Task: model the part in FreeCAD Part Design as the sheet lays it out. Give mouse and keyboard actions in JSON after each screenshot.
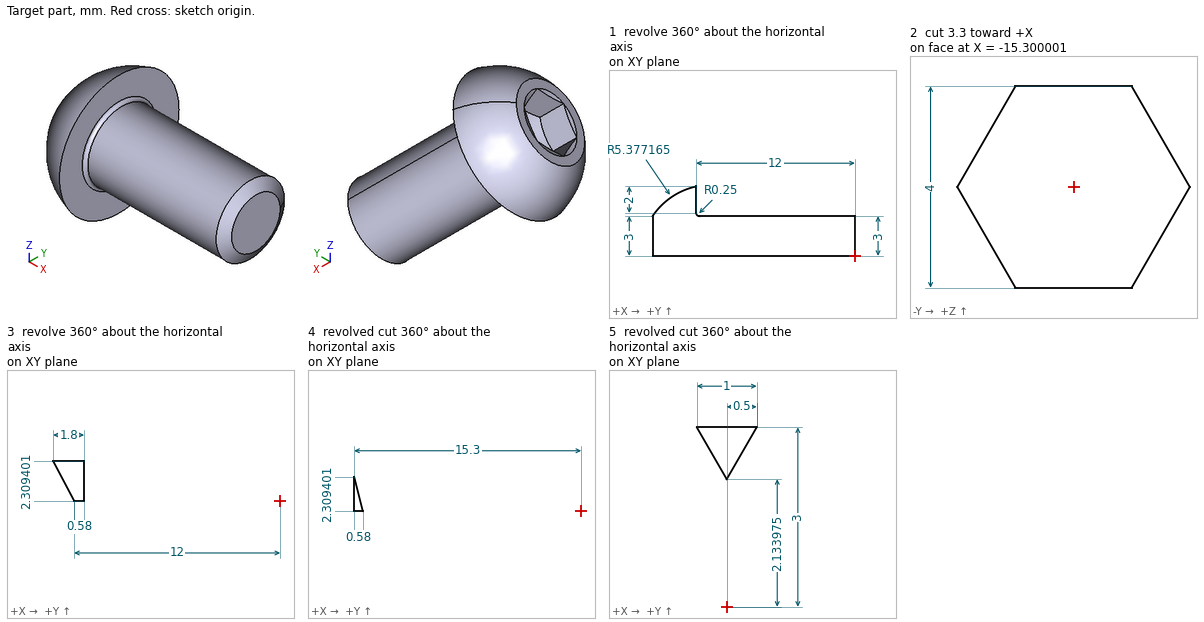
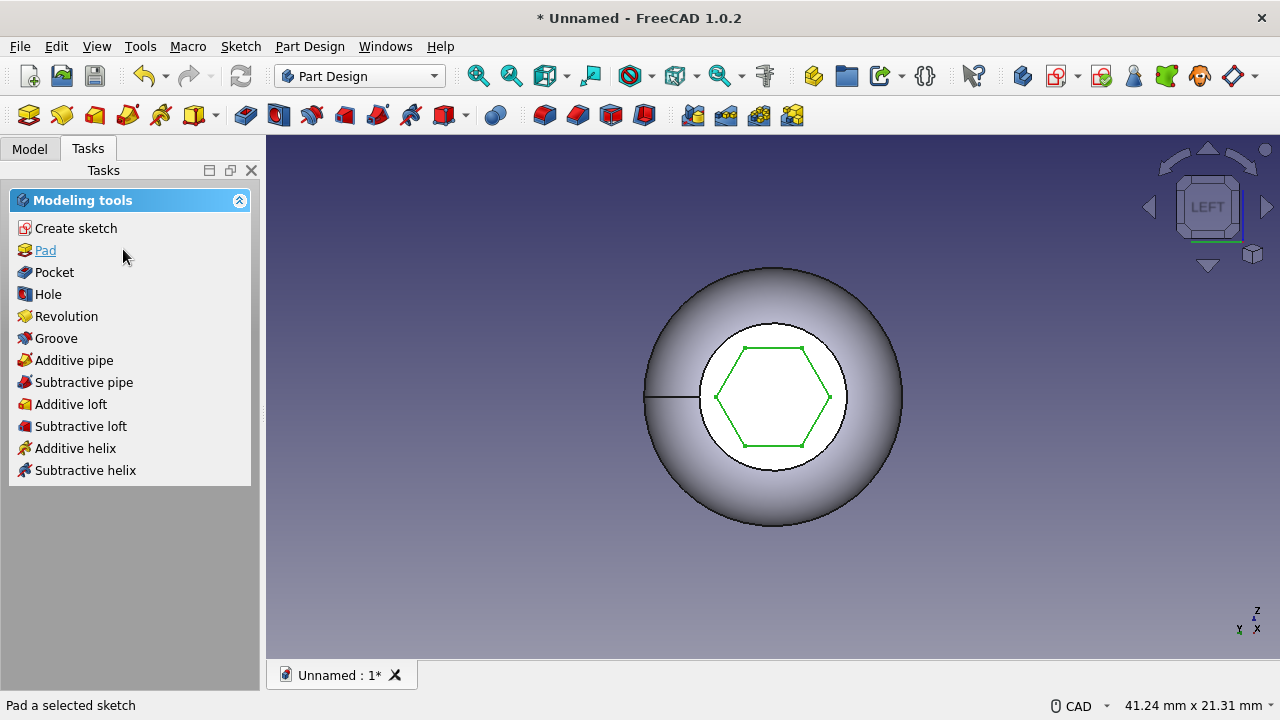
{"action": "left_click", "coordinate": [246, 116]}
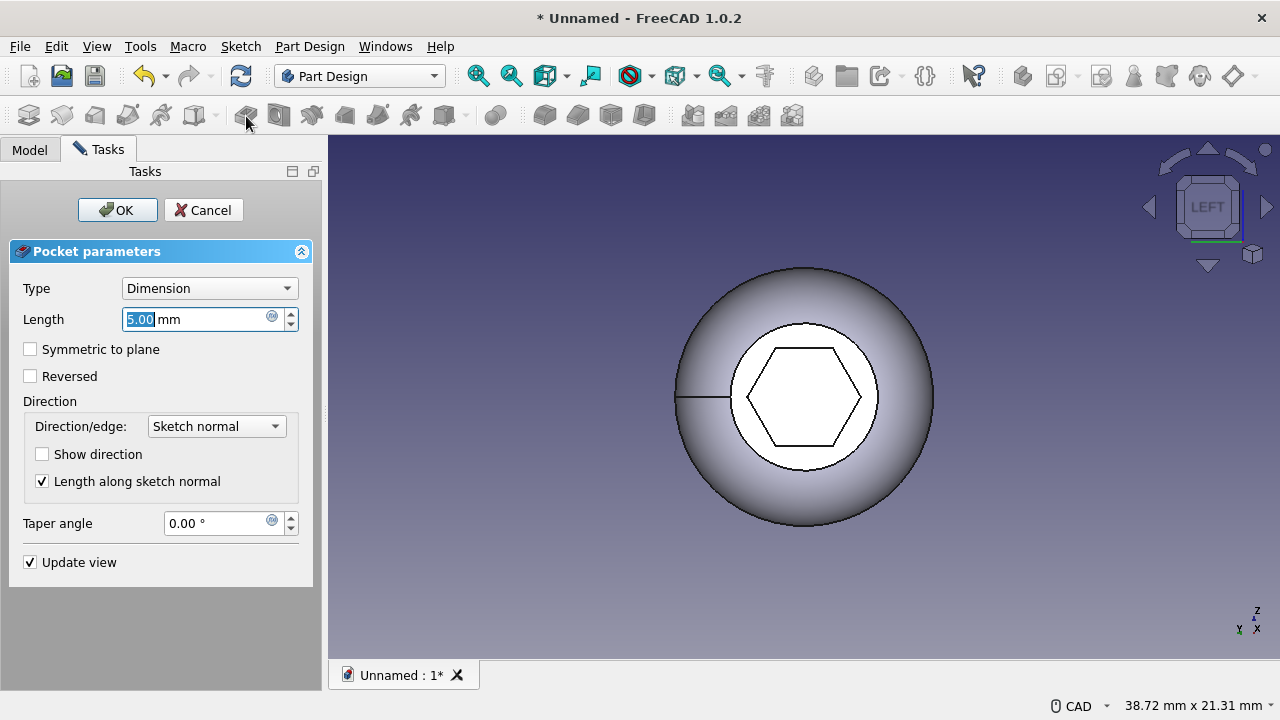
{"action": "type", "text": "3.3"}
{"action": "key", "text": "Tab"}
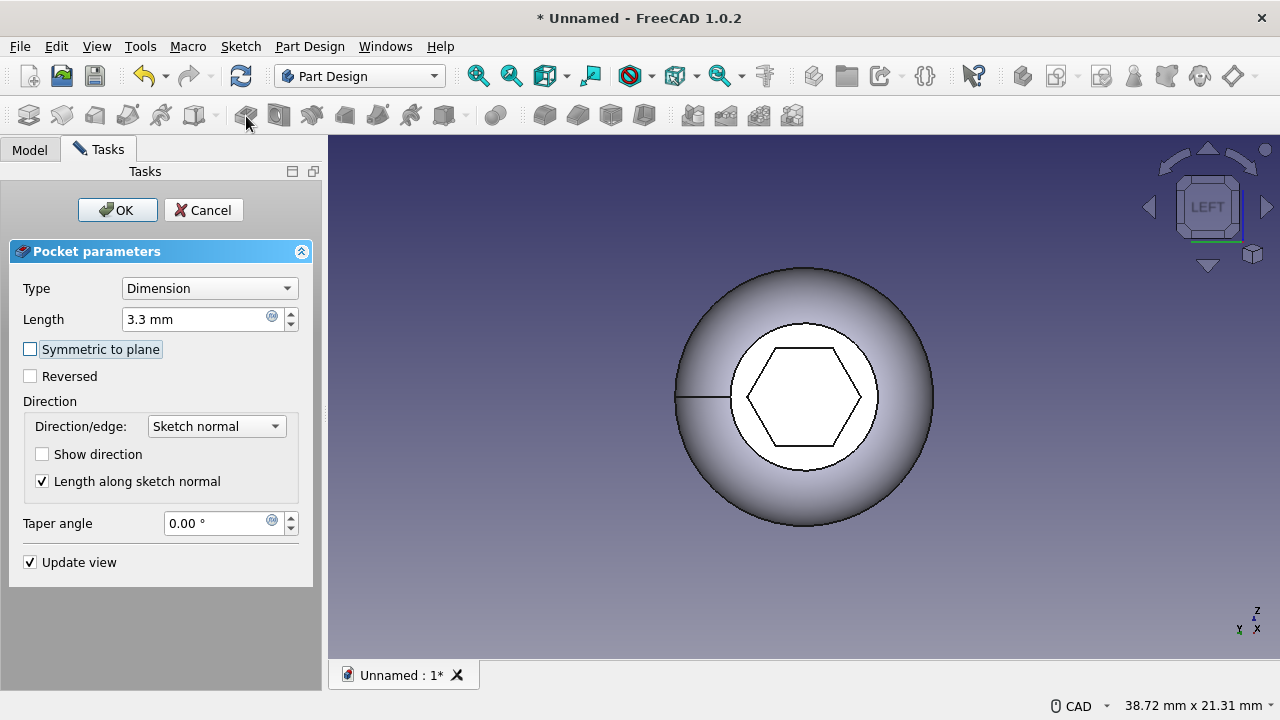
{"action": "left_click", "coordinate": [118, 210]}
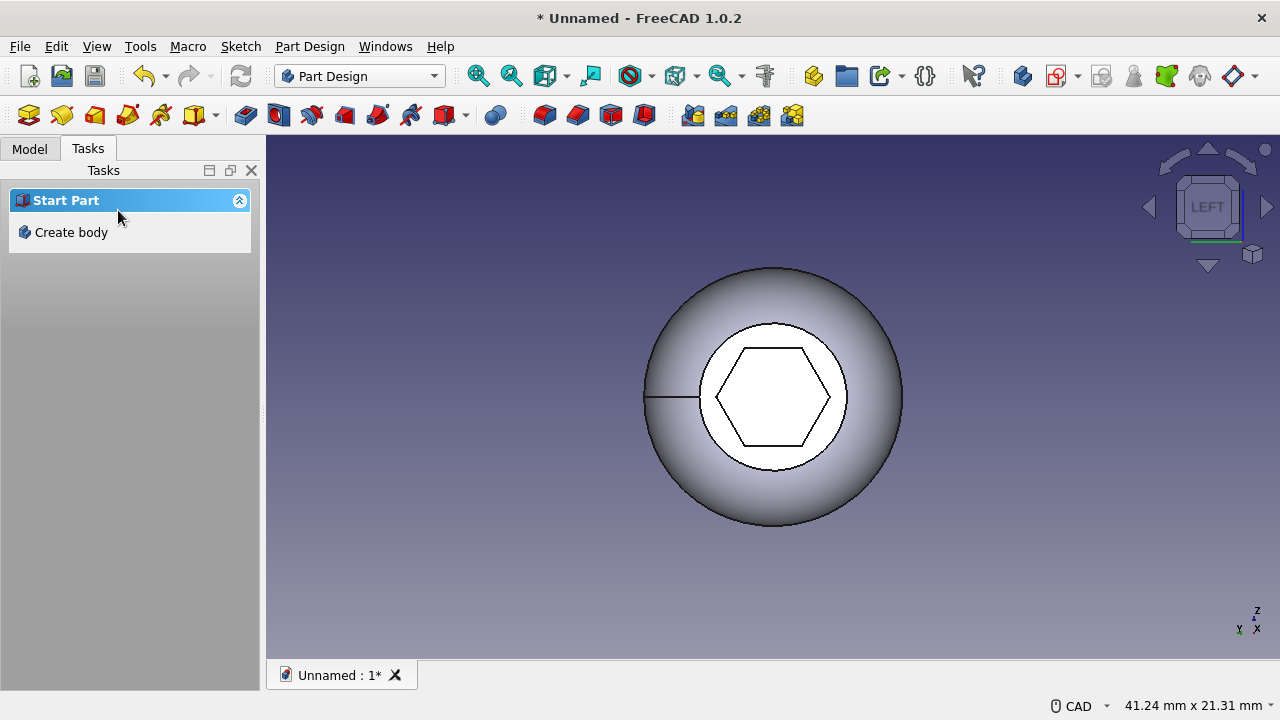
{"action": "left_click", "coordinate": [1056, 76]}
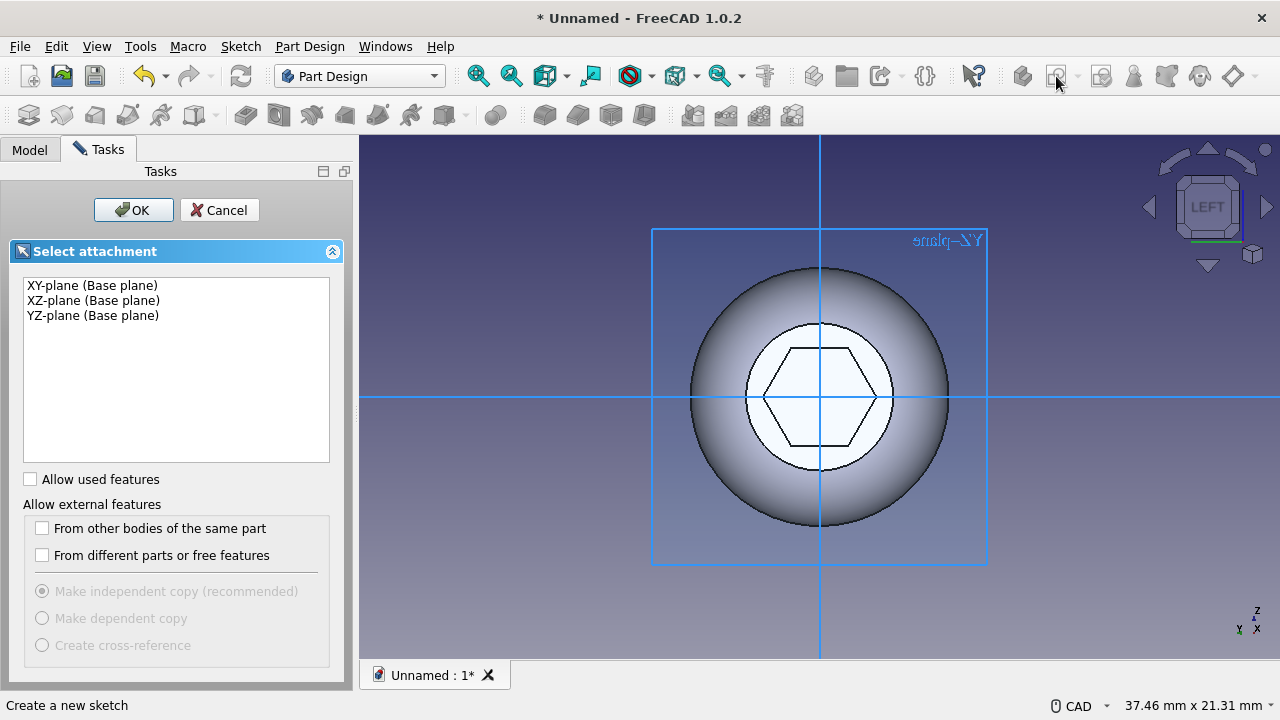
{"action": "left_click", "coordinate": [84, 286]}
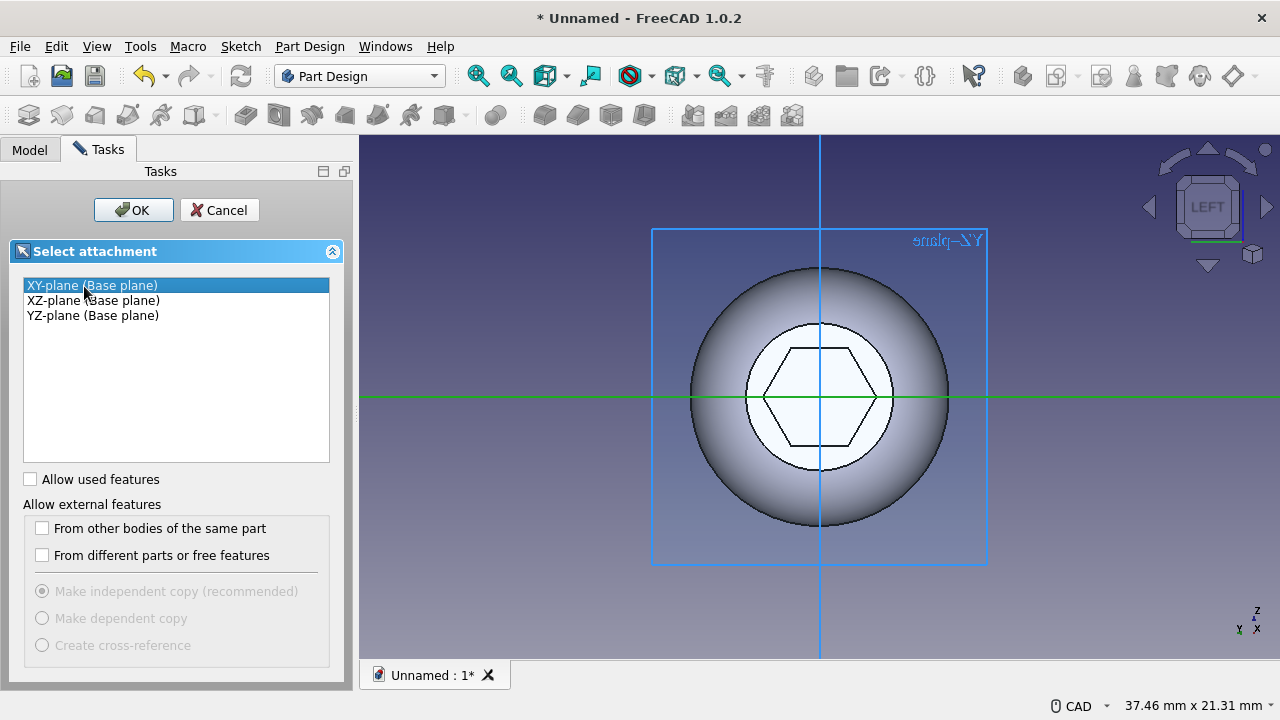
{"action": "left_click", "coordinate": [134, 210]}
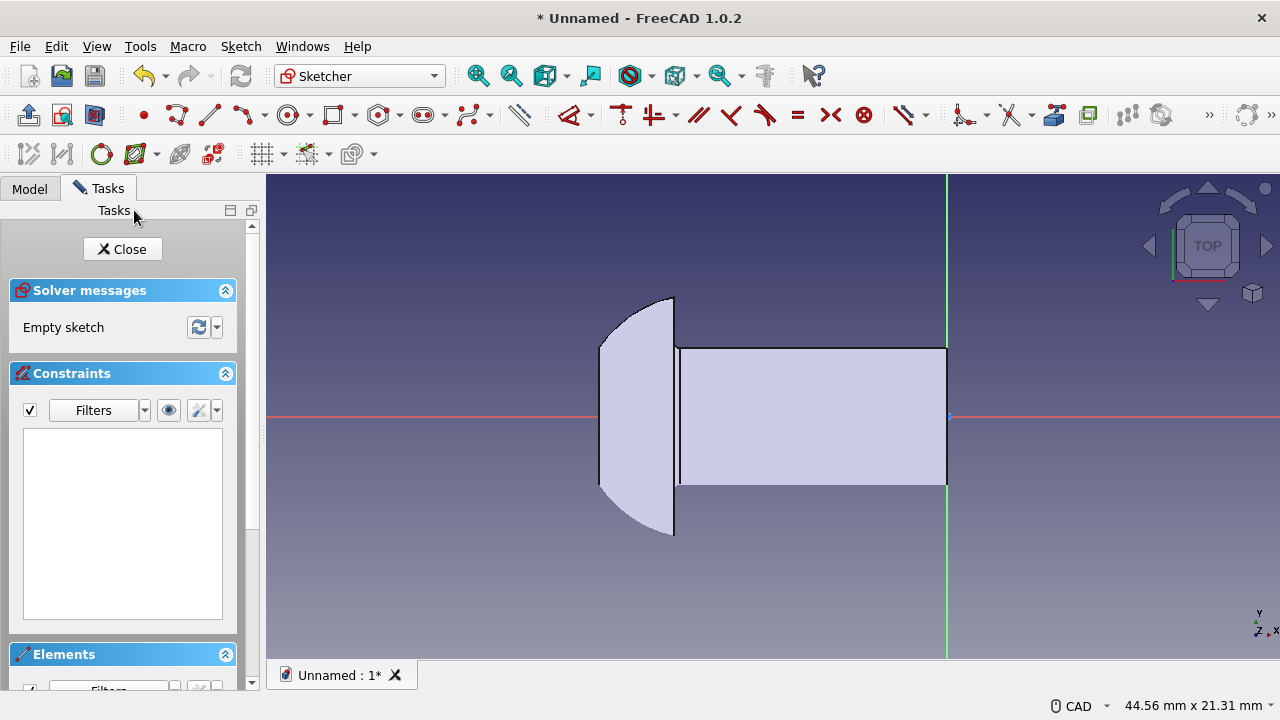
{"action": "key", "text": "q s"}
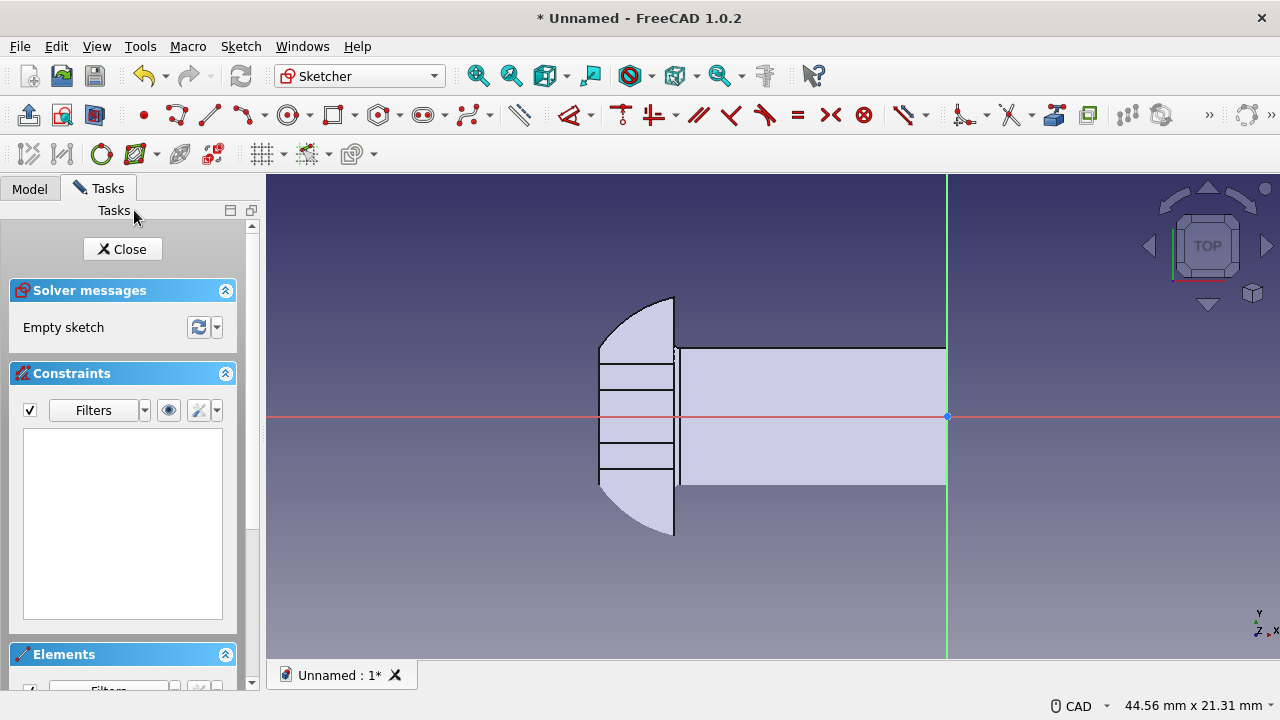
{"action": "scroll", "coordinate": [659, 385], "scroll_direction": "up", "scroll_amount": 9}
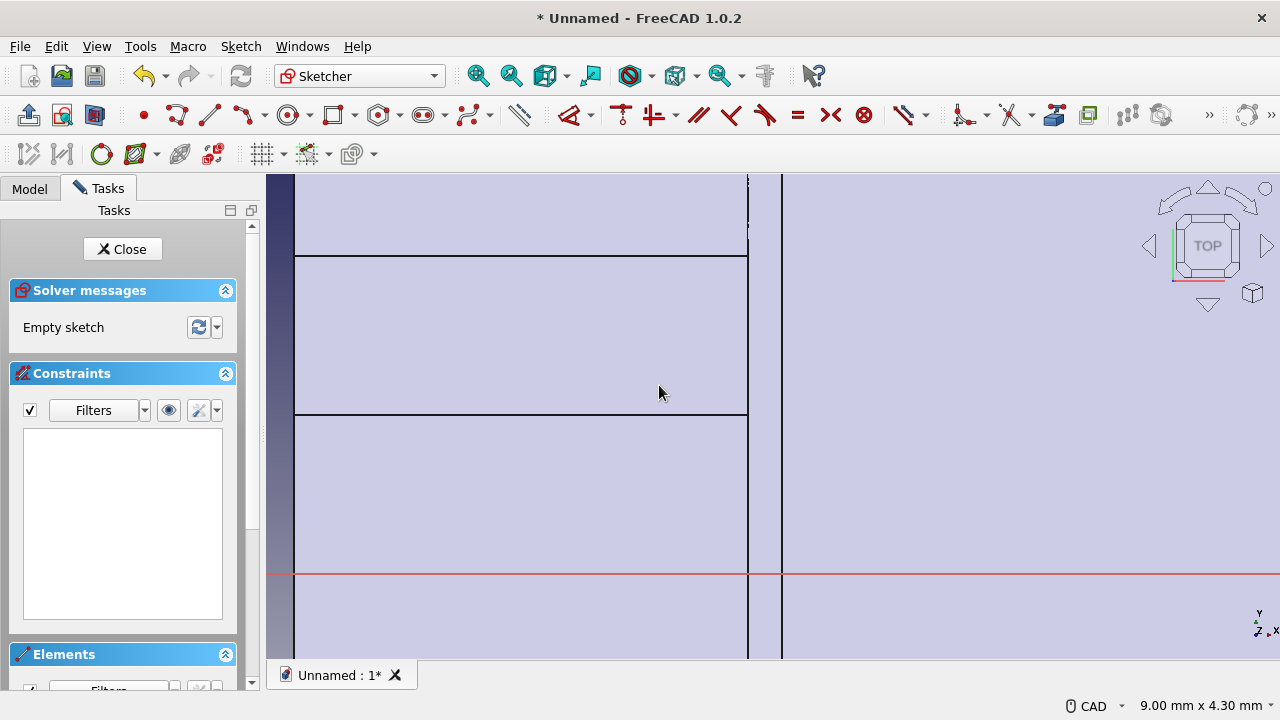
{"action": "left_click", "coordinate": [177, 116]}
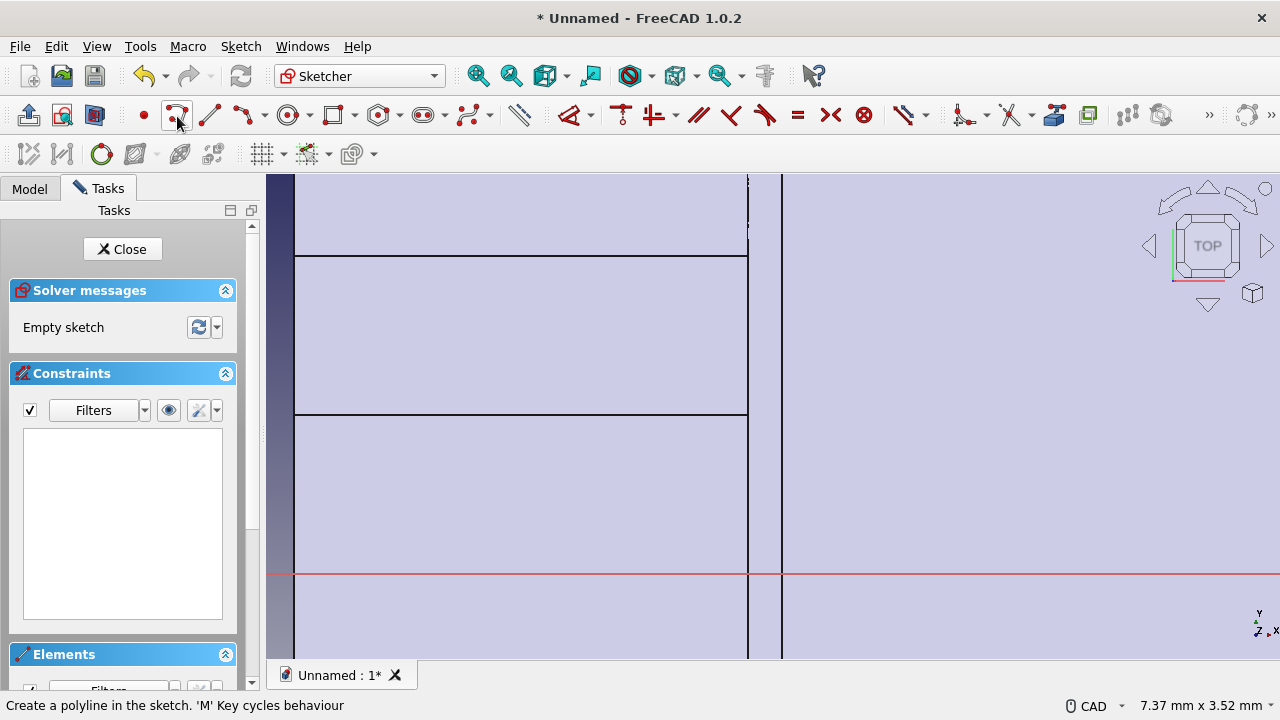
{"action": "left_click", "coordinate": [828, 574]}
{"action": "left_click", "coordinate": [828, 256]}
{"action": "left_click", "coordinate": [580, 256]}
{"action": "left_click", "coordinate": [748, 565]}
{"action": "left_click", "coordinate": [828, 574]}
{"action": "key", "text": "Escape"}
{"action": "key", "text": "Escape"}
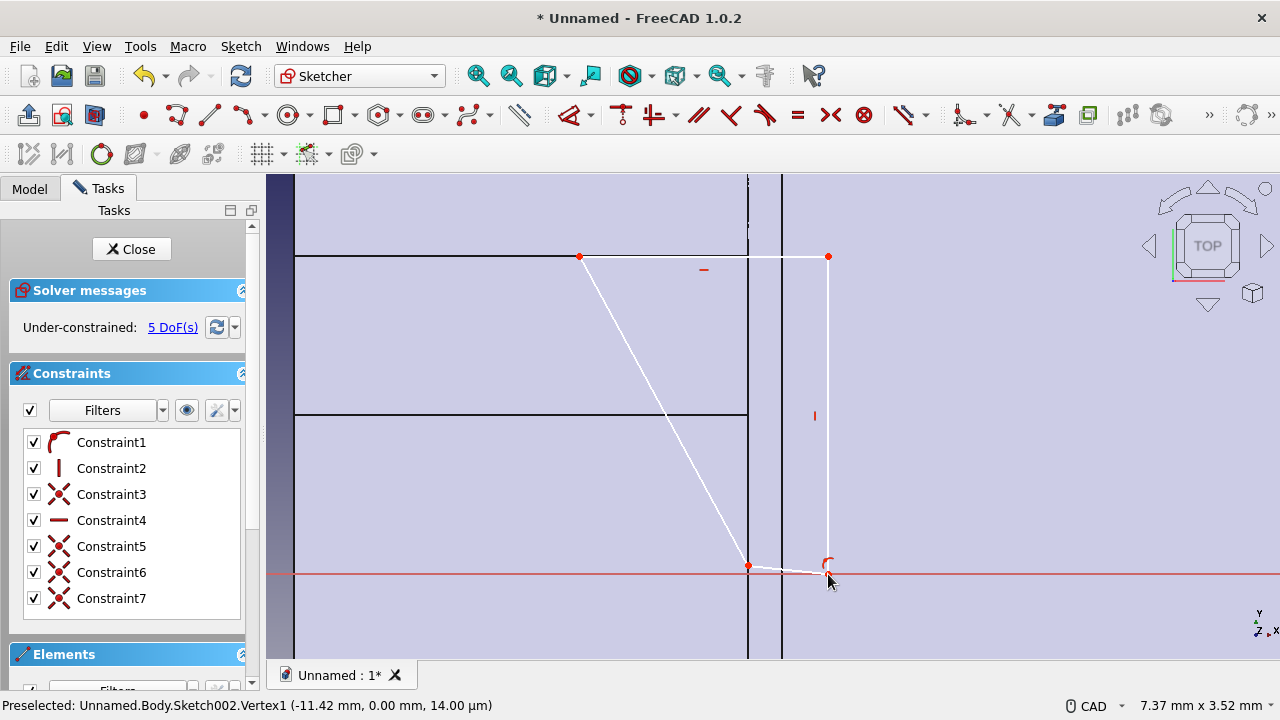
{"action": "left_click", "coordinate": [804, 572]}